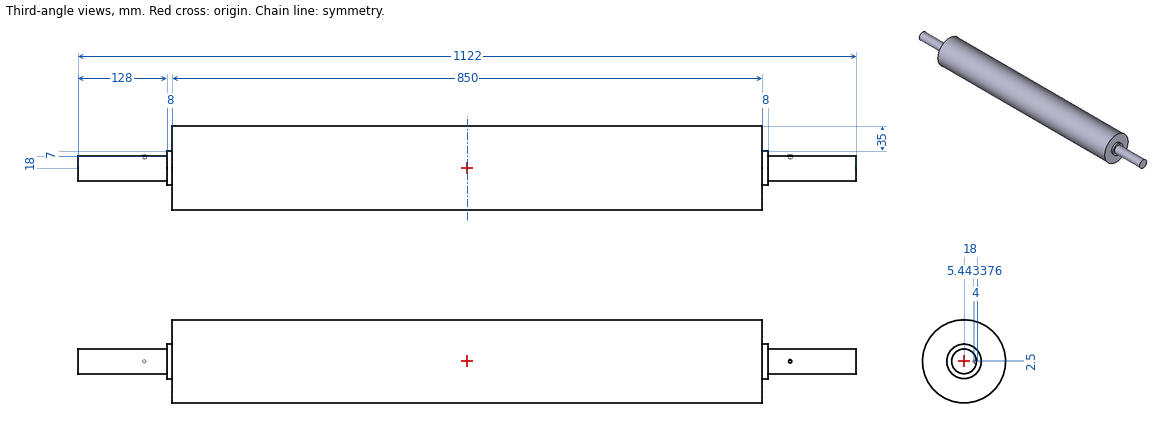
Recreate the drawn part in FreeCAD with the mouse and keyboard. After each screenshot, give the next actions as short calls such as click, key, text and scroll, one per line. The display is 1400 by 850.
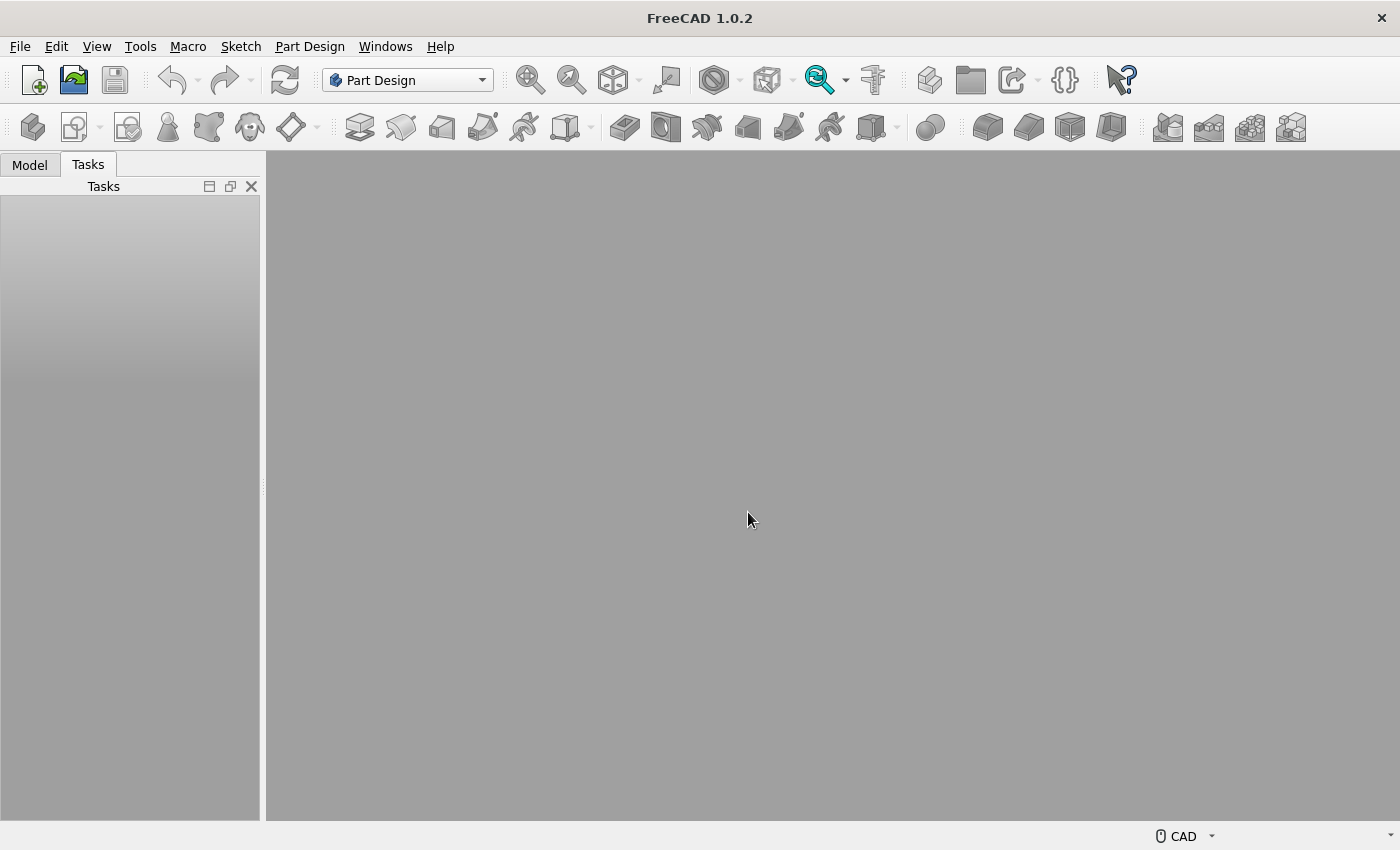
click(33, 80)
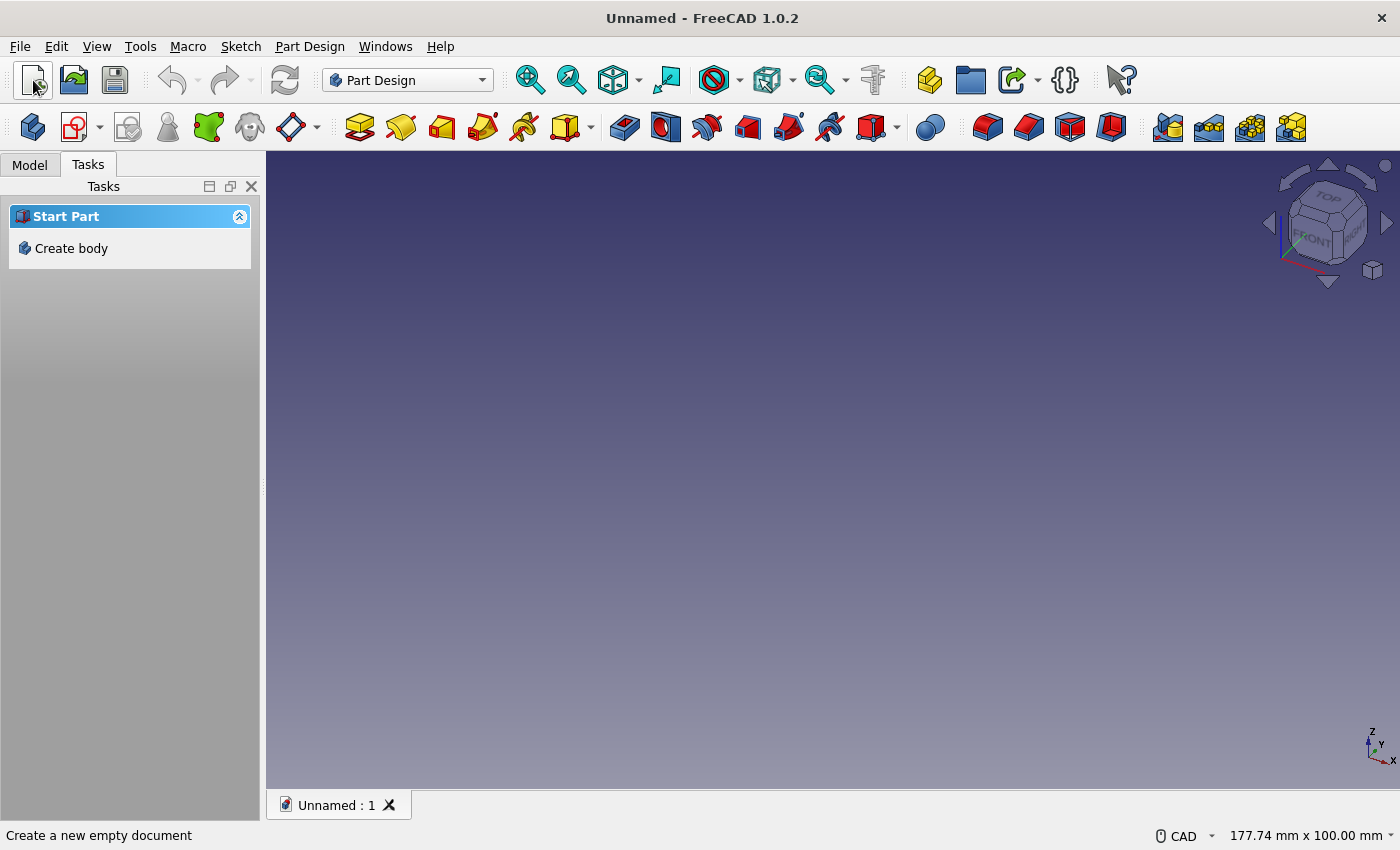
click(74, 128)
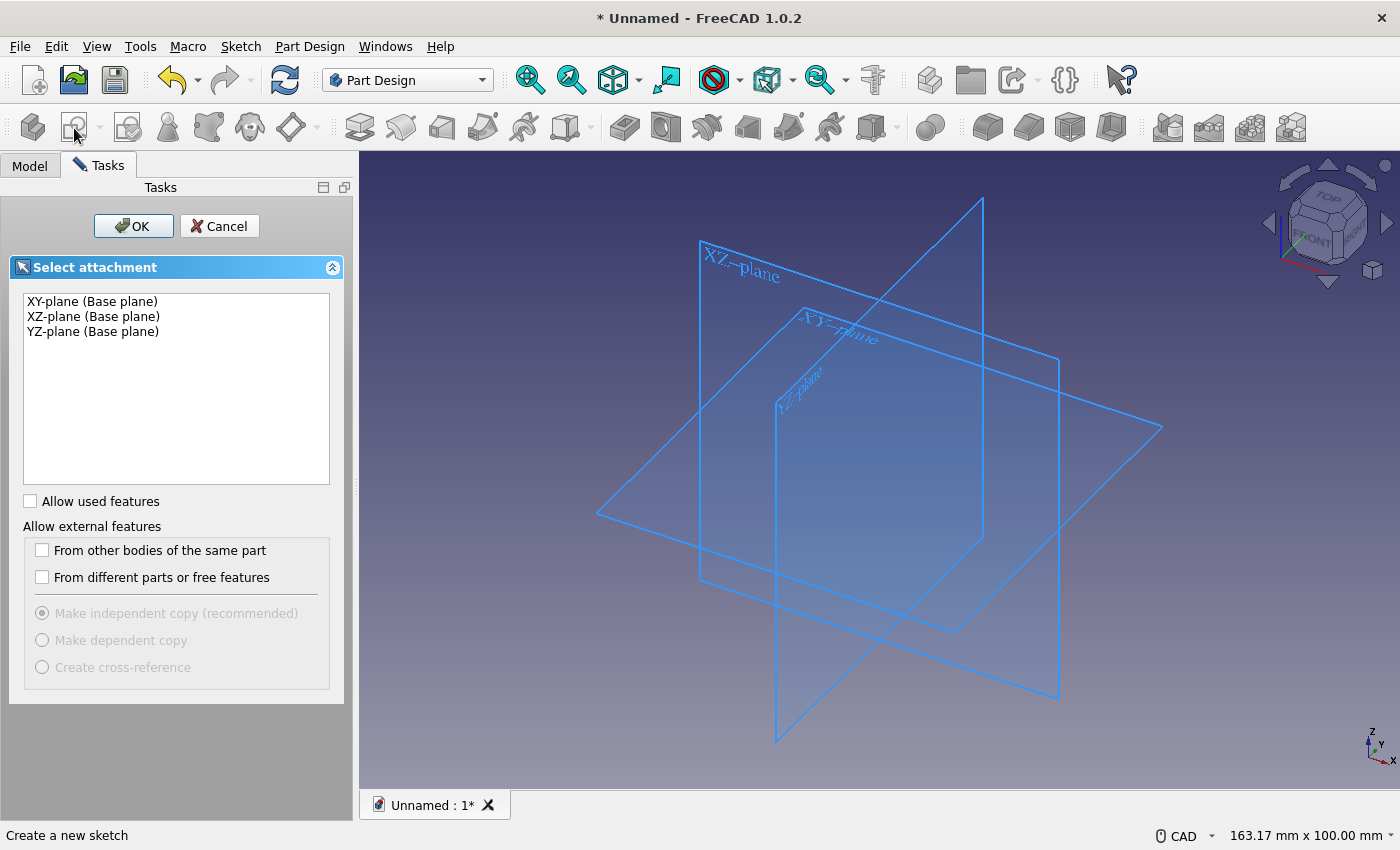
click(84, 302)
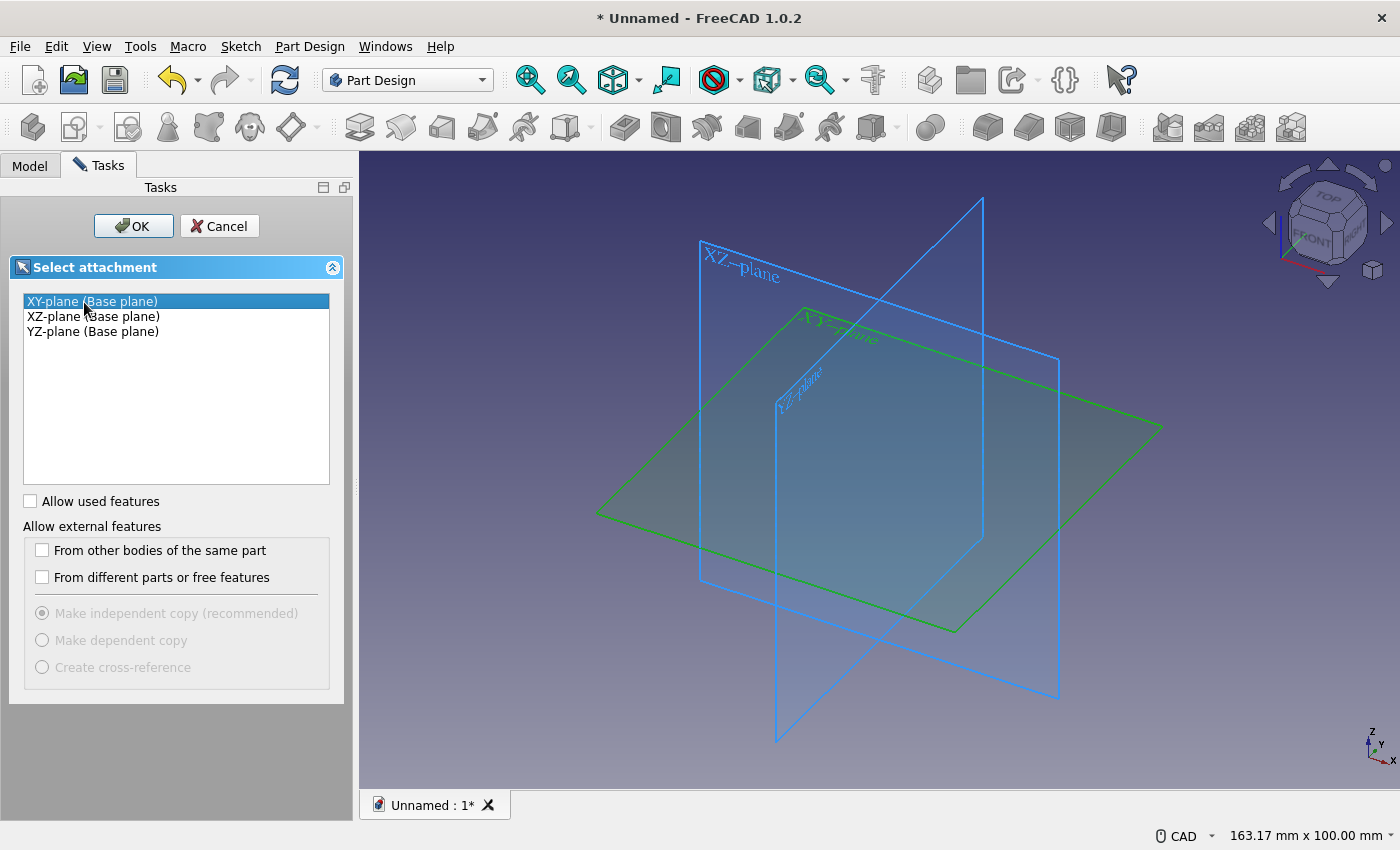
click(134, 226)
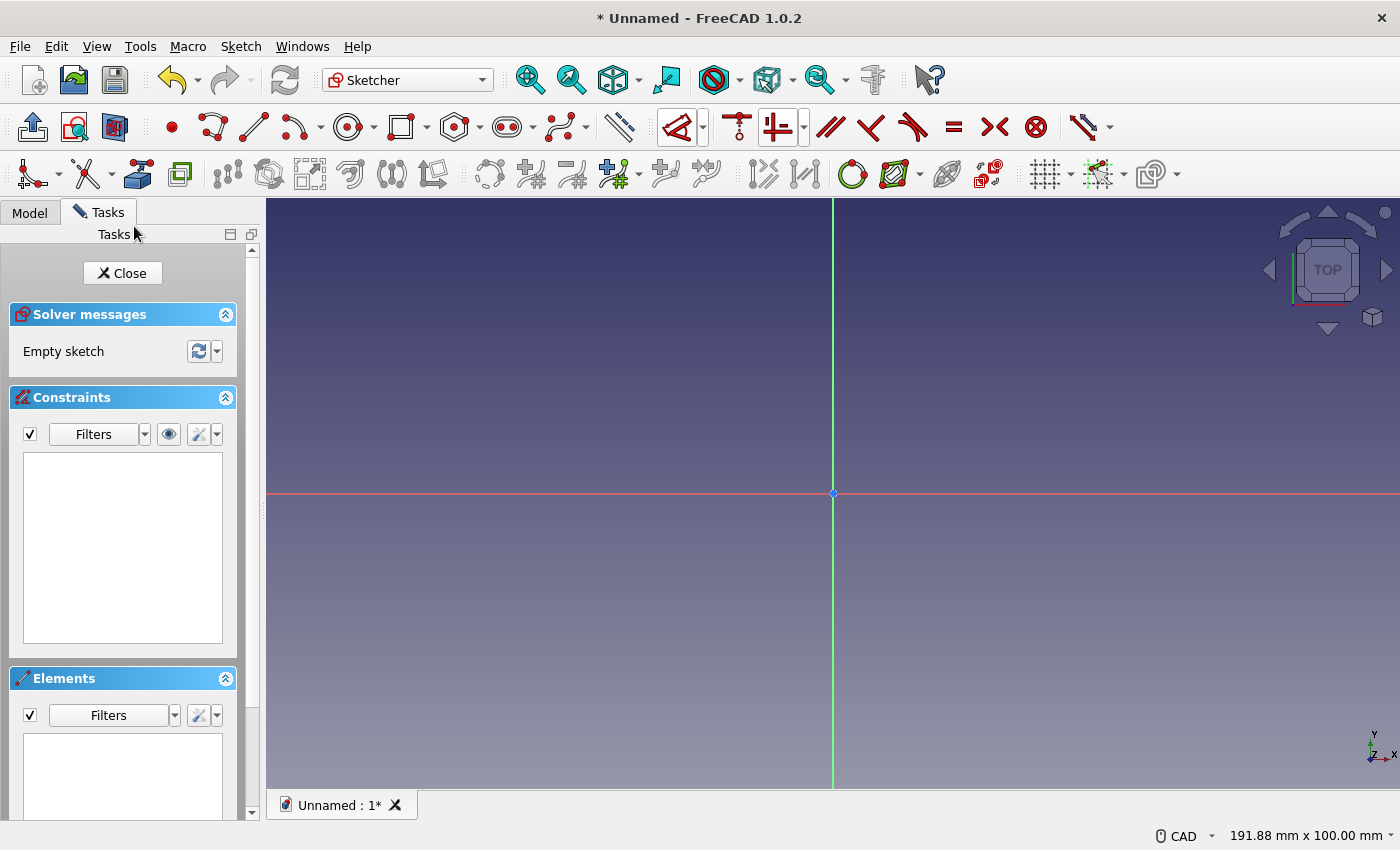
scroll(758, 511, down, 12)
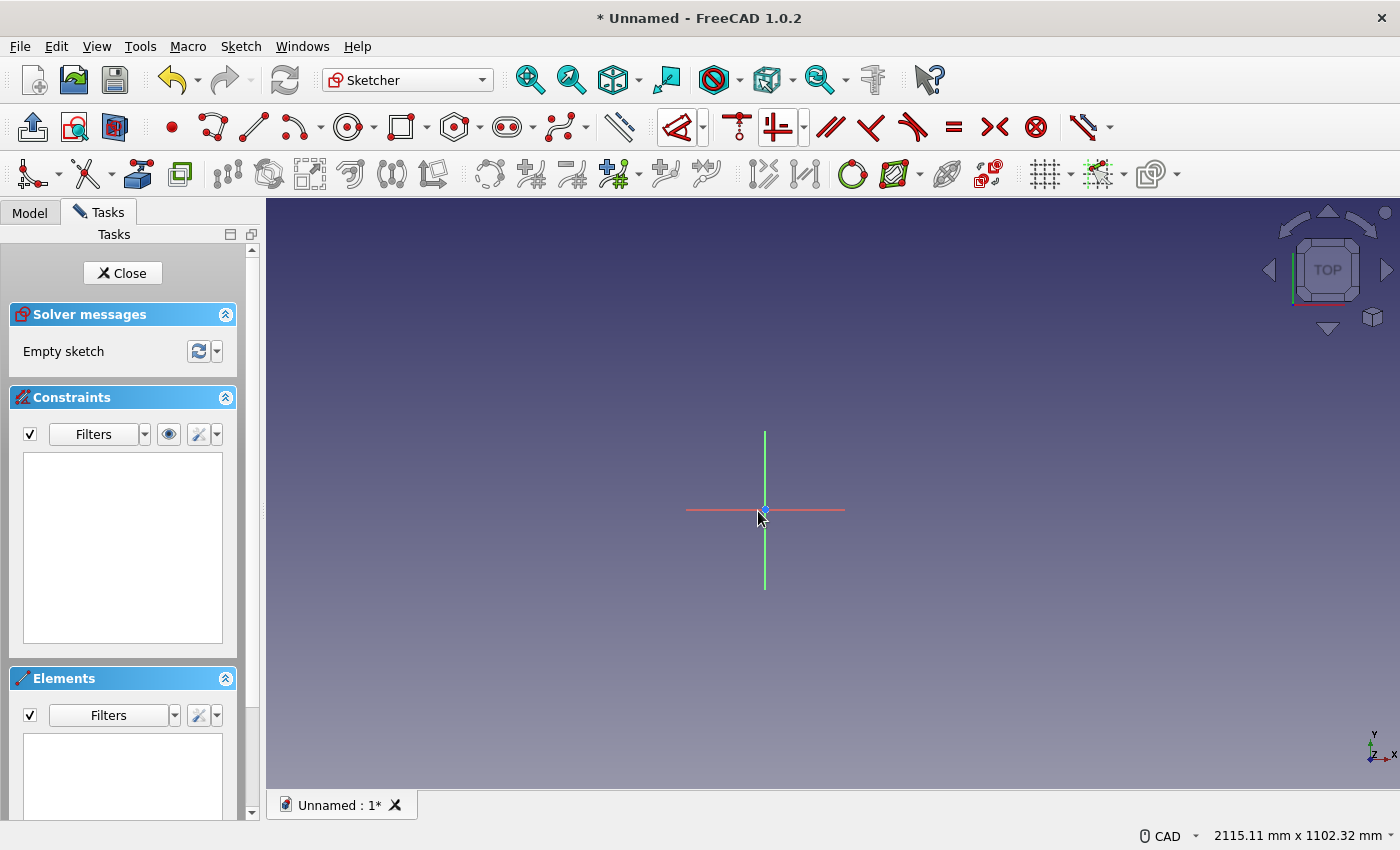
key(g)
key(m)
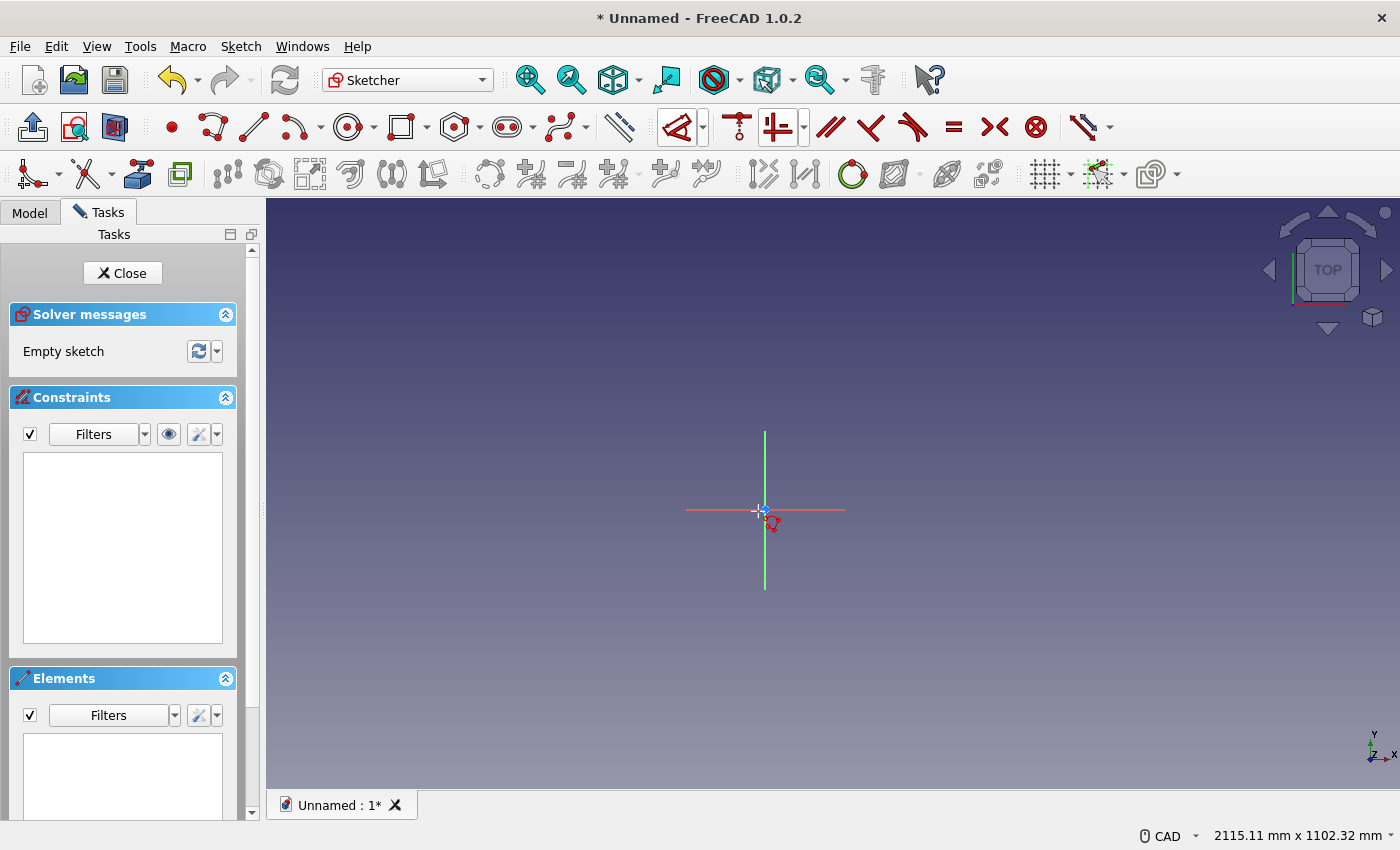
click(537, 496)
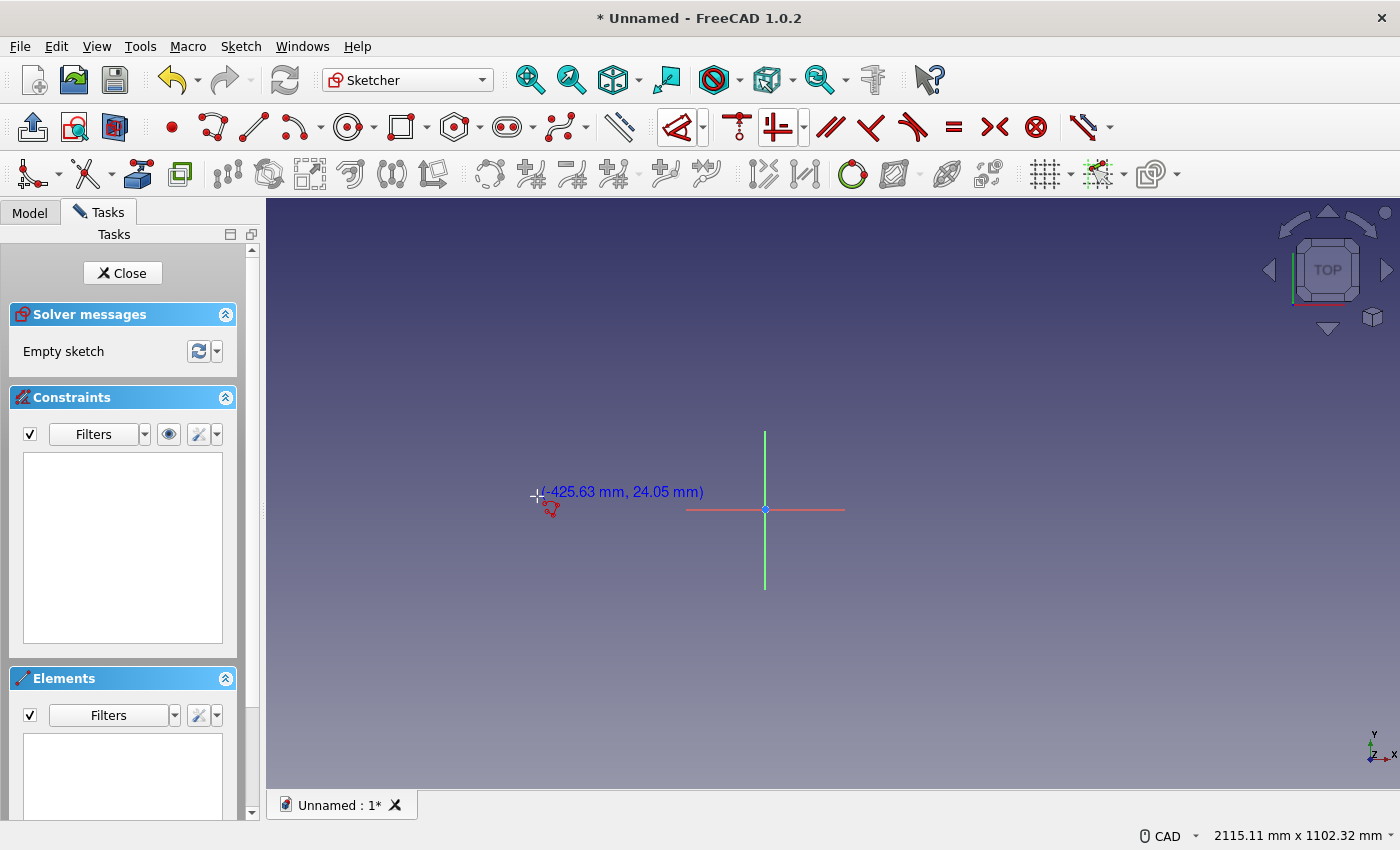
scroll(533, 496, up, 7)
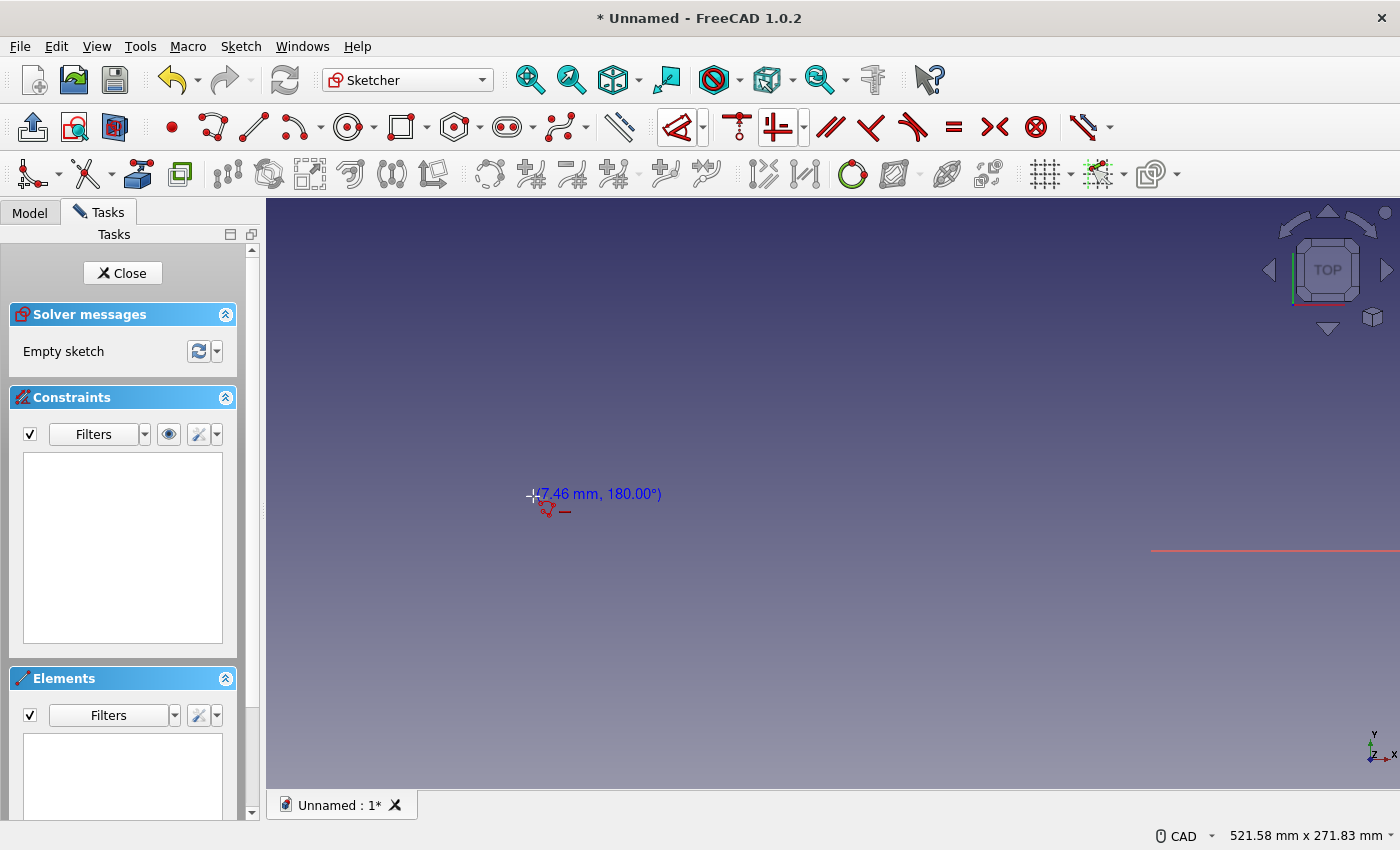
click(532, 494)
click(532, 512)